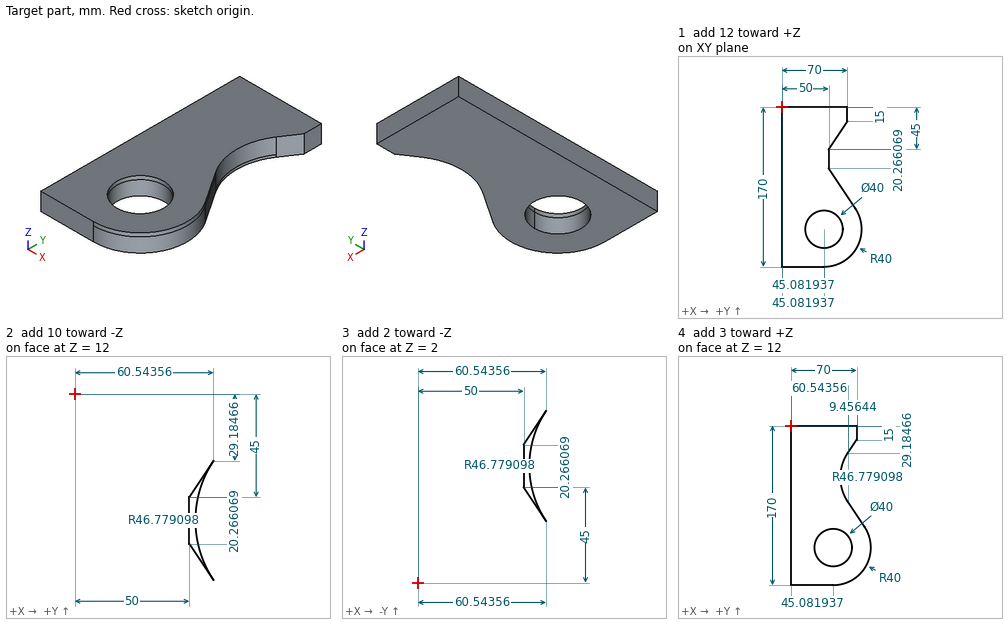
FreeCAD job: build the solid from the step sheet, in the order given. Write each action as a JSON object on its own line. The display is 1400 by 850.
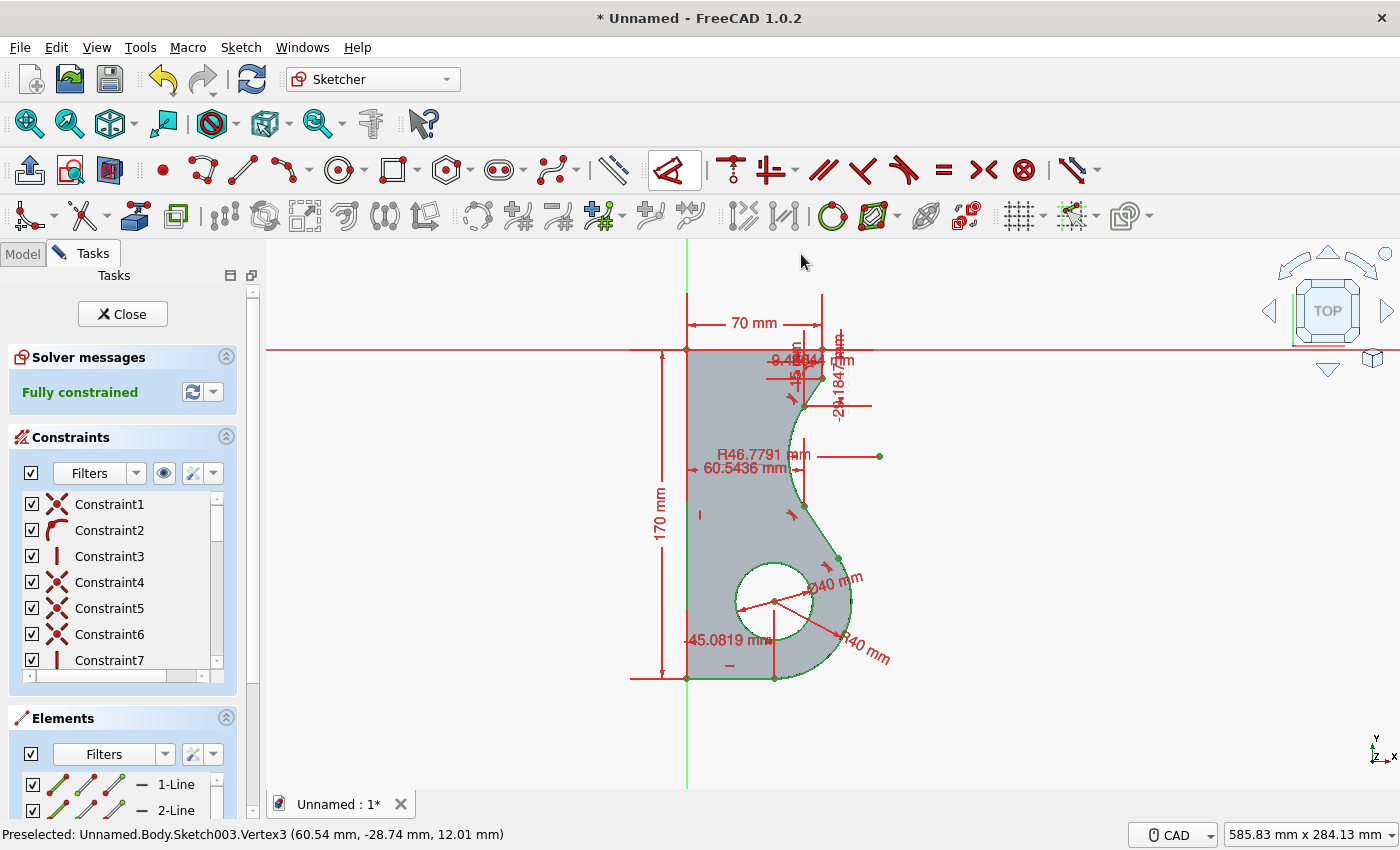
{"action": "left_click", "coordinate": [123, 314]}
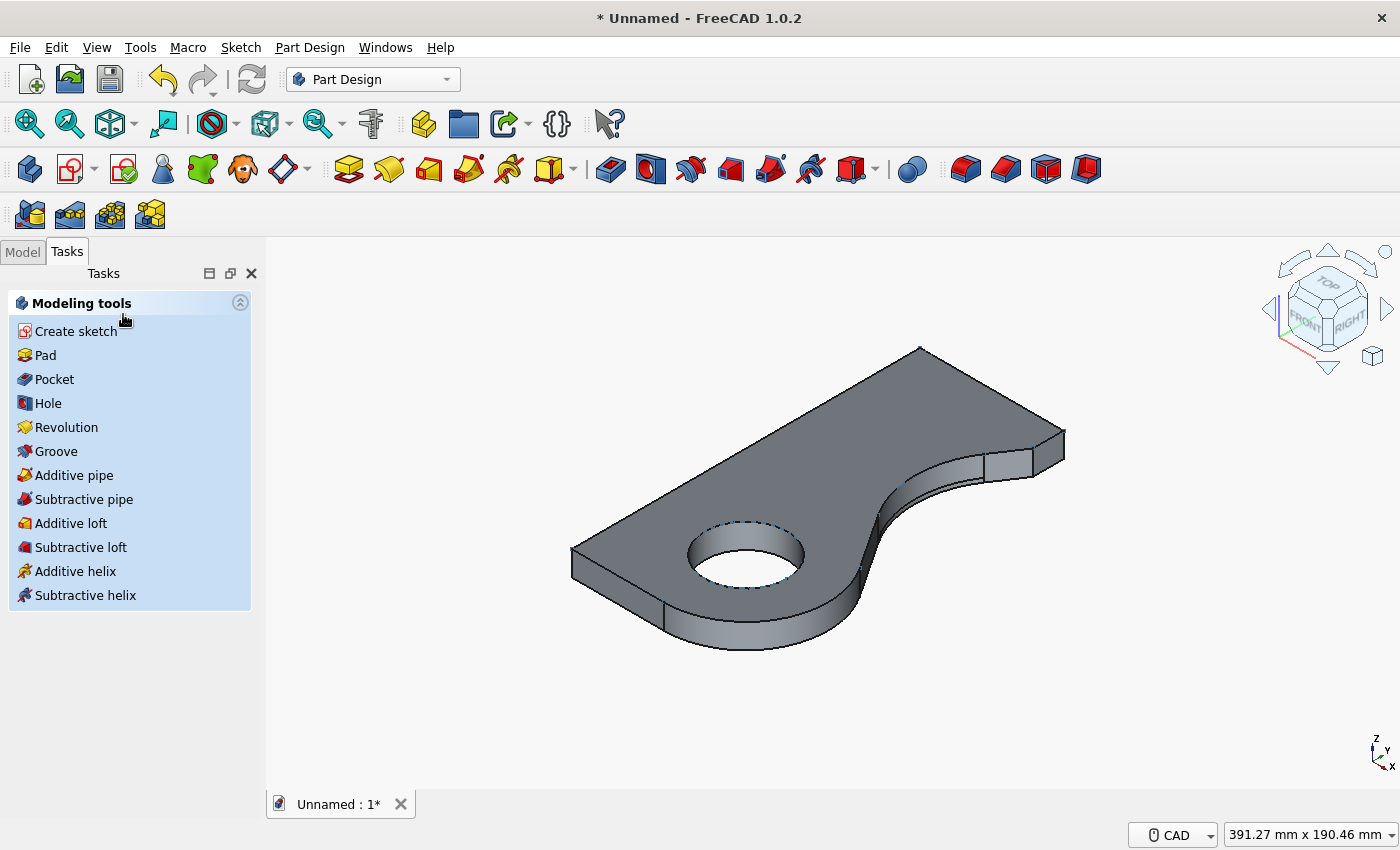
{"action": "left_click", "coordinate": [350, 170]}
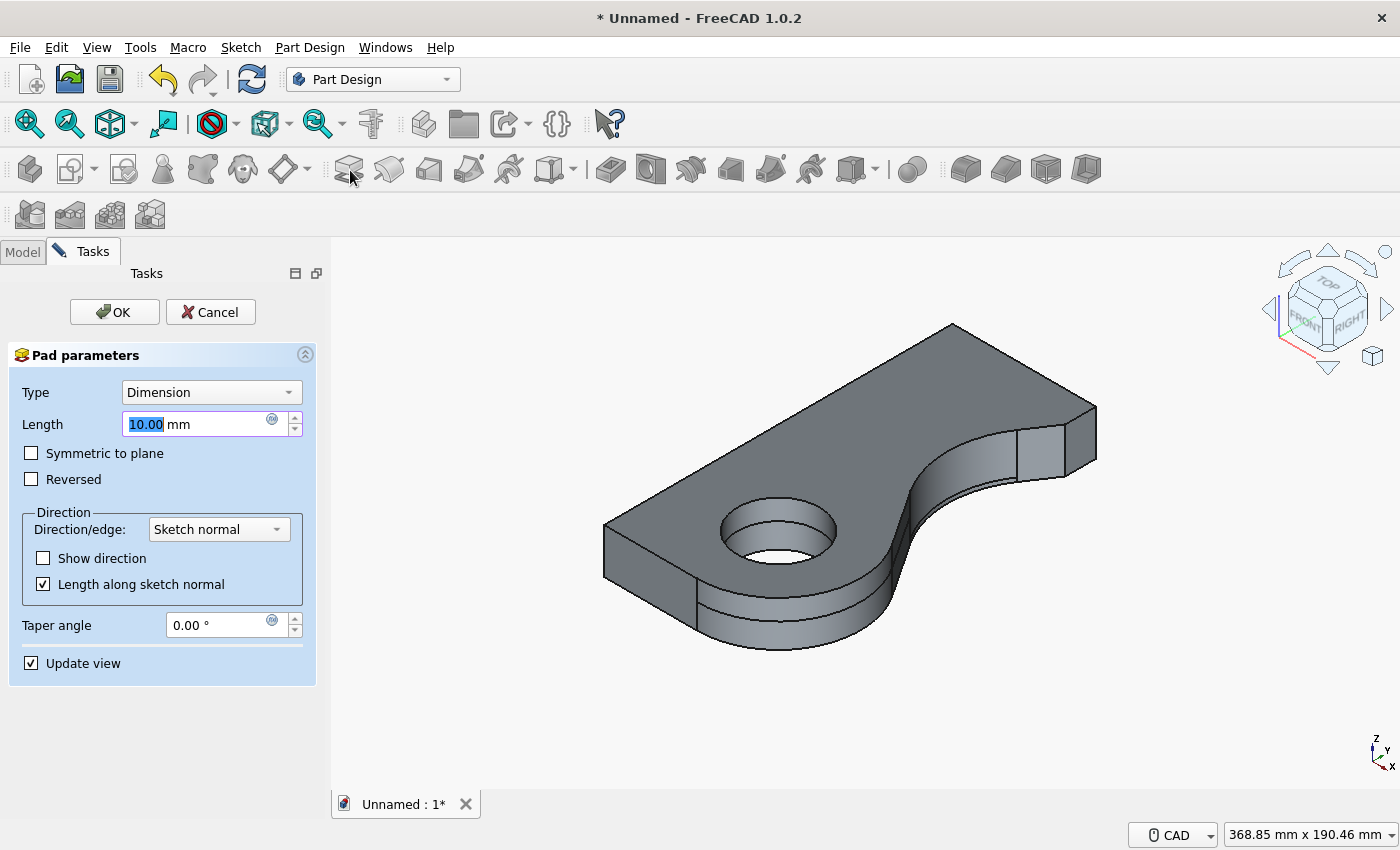
{"action": "type", "text": "3"}
{"action": "key", "text": "Tab"}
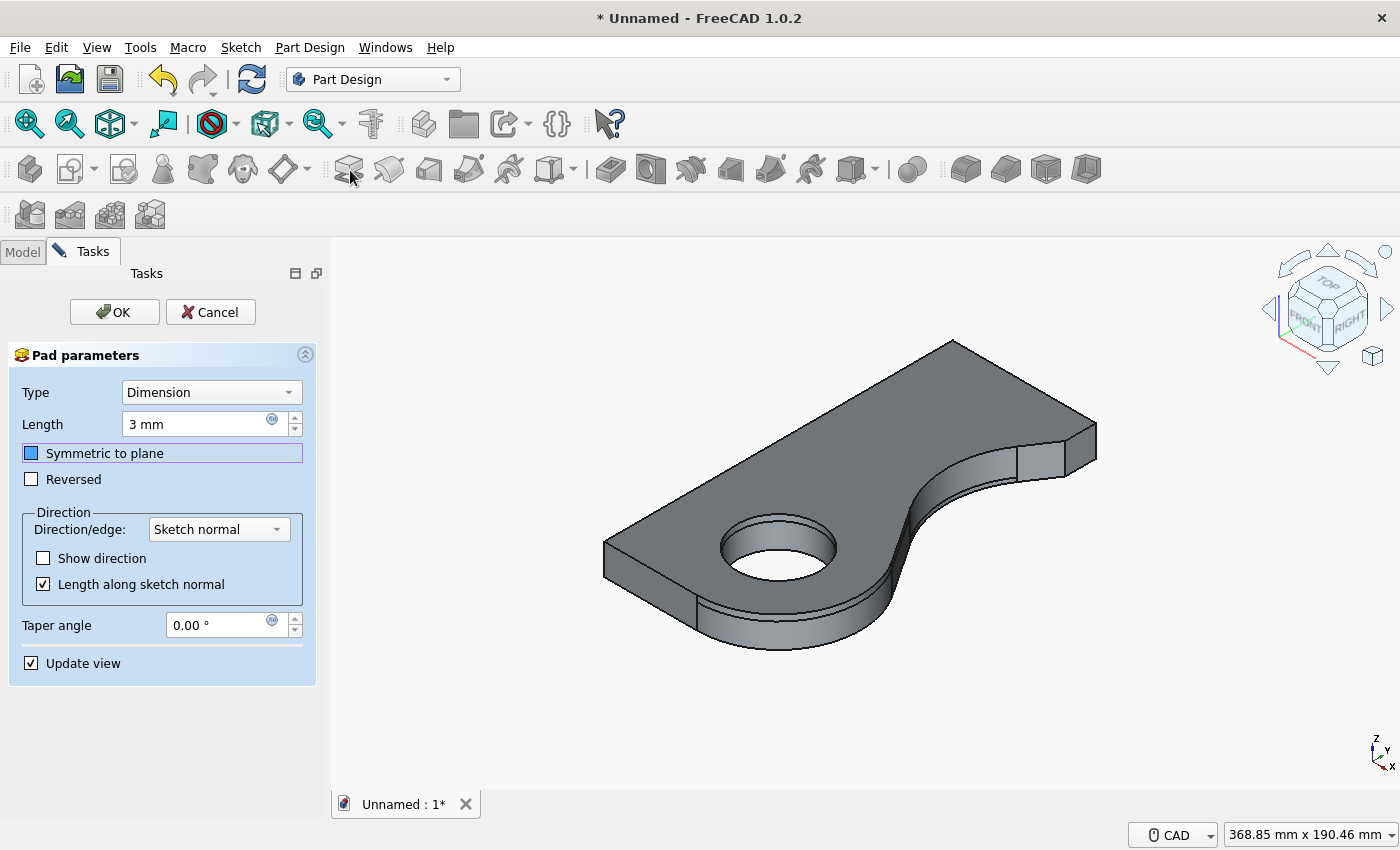
{"action": "left_click", "coordinate": [115, 312]}